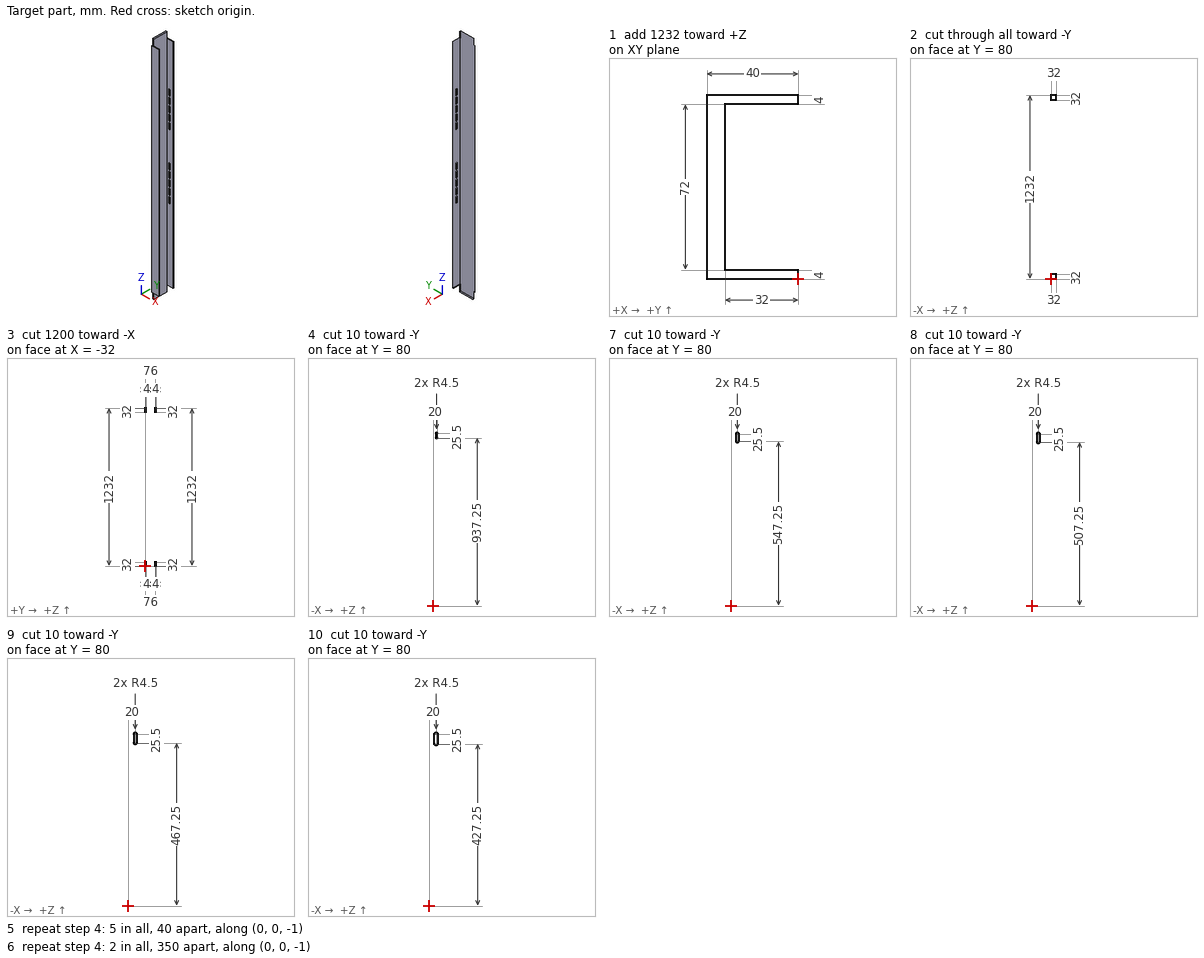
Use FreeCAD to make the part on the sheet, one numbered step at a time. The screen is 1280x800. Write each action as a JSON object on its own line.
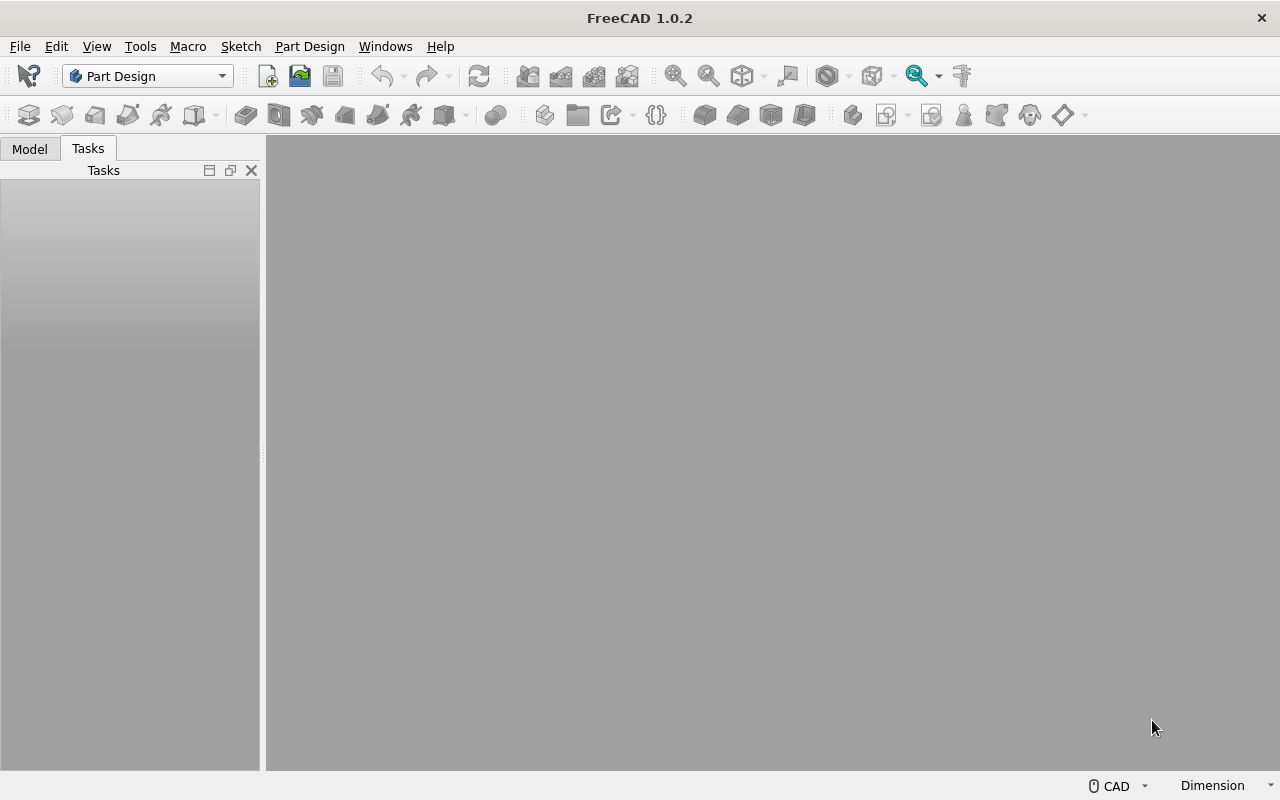
{"action": "left_click", "coordinate": [267, 76]}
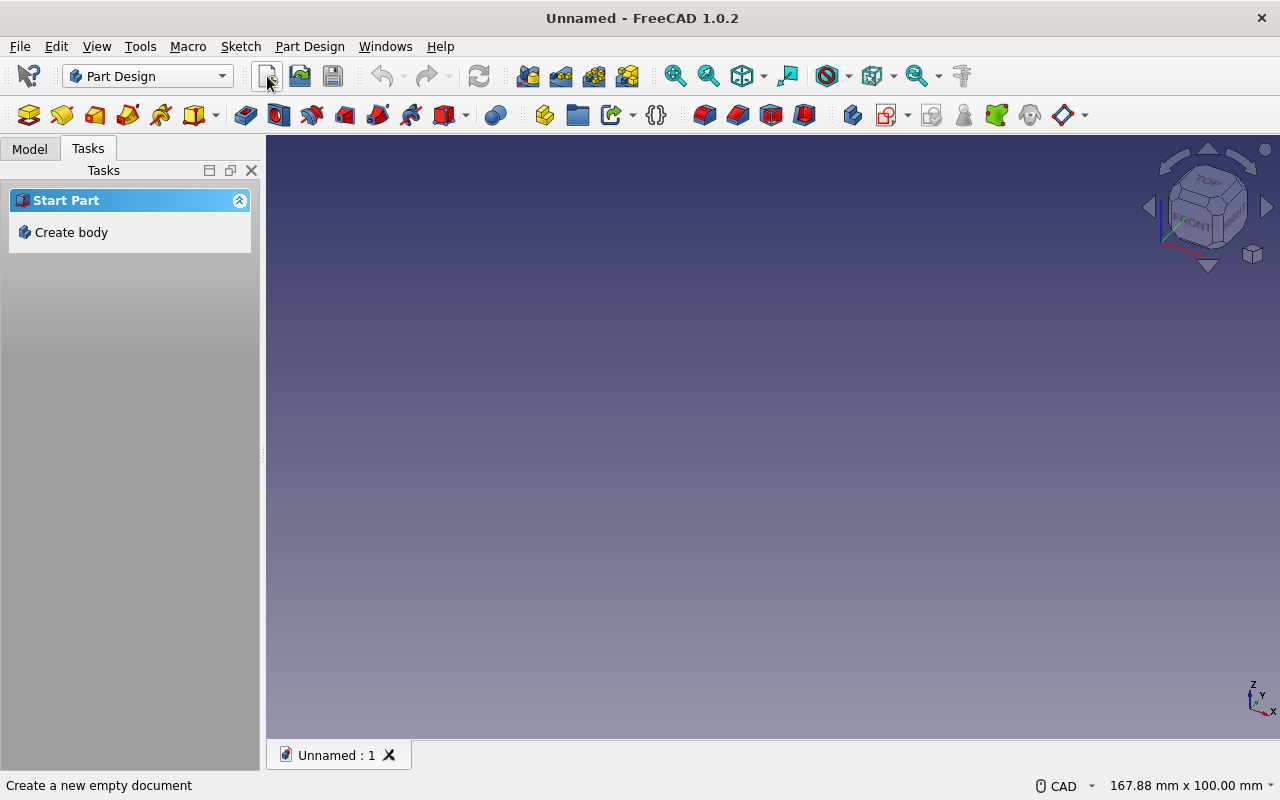
{"action": "left_click", "coordinate": [886, 116]}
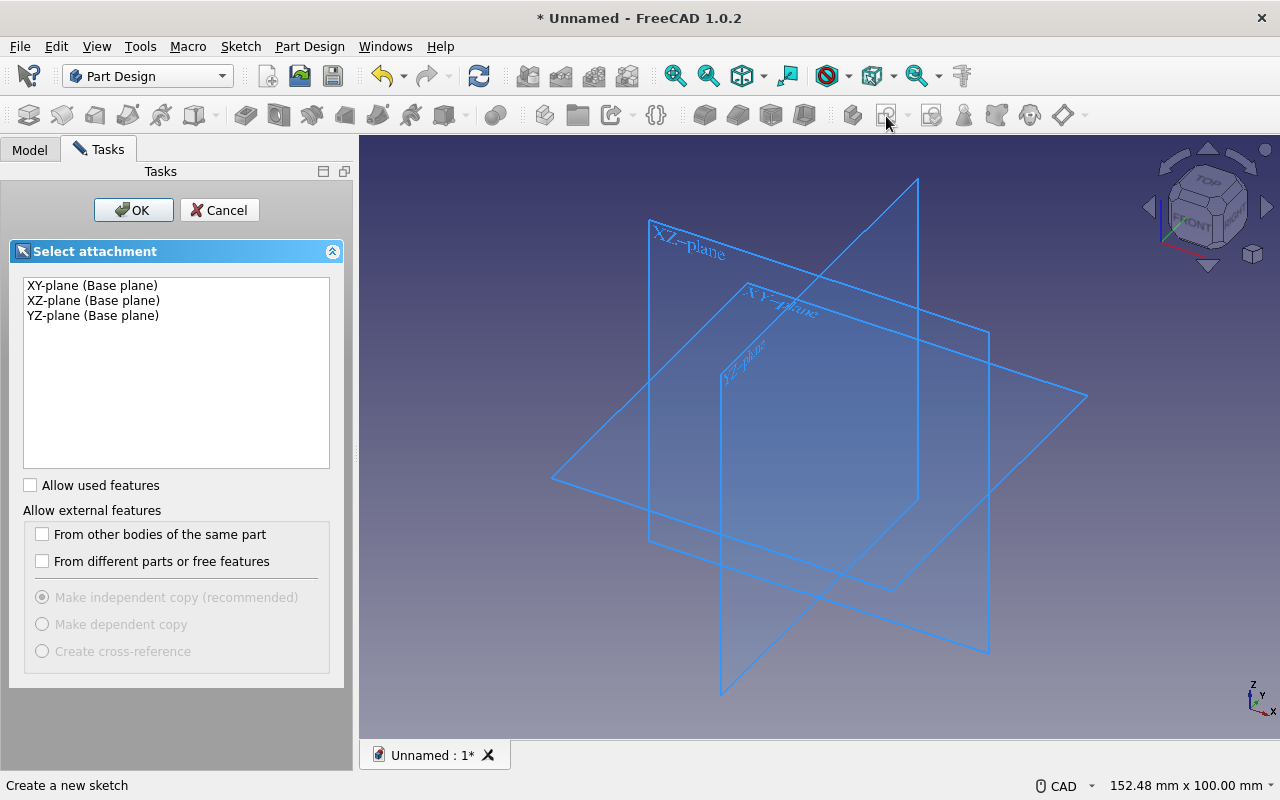
{"action": "left_click", "coordinate": [84, 286]}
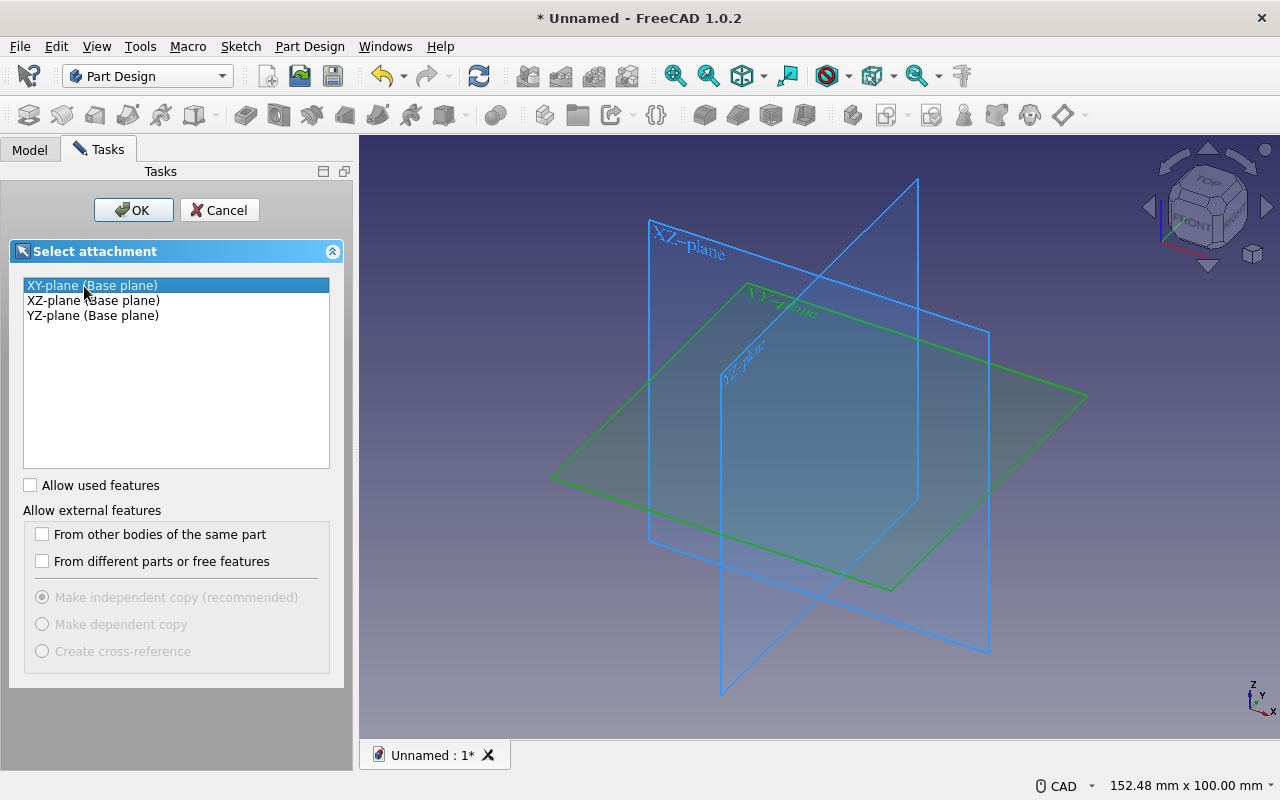
{"action": "left_click", "coordinate": [134, 210]}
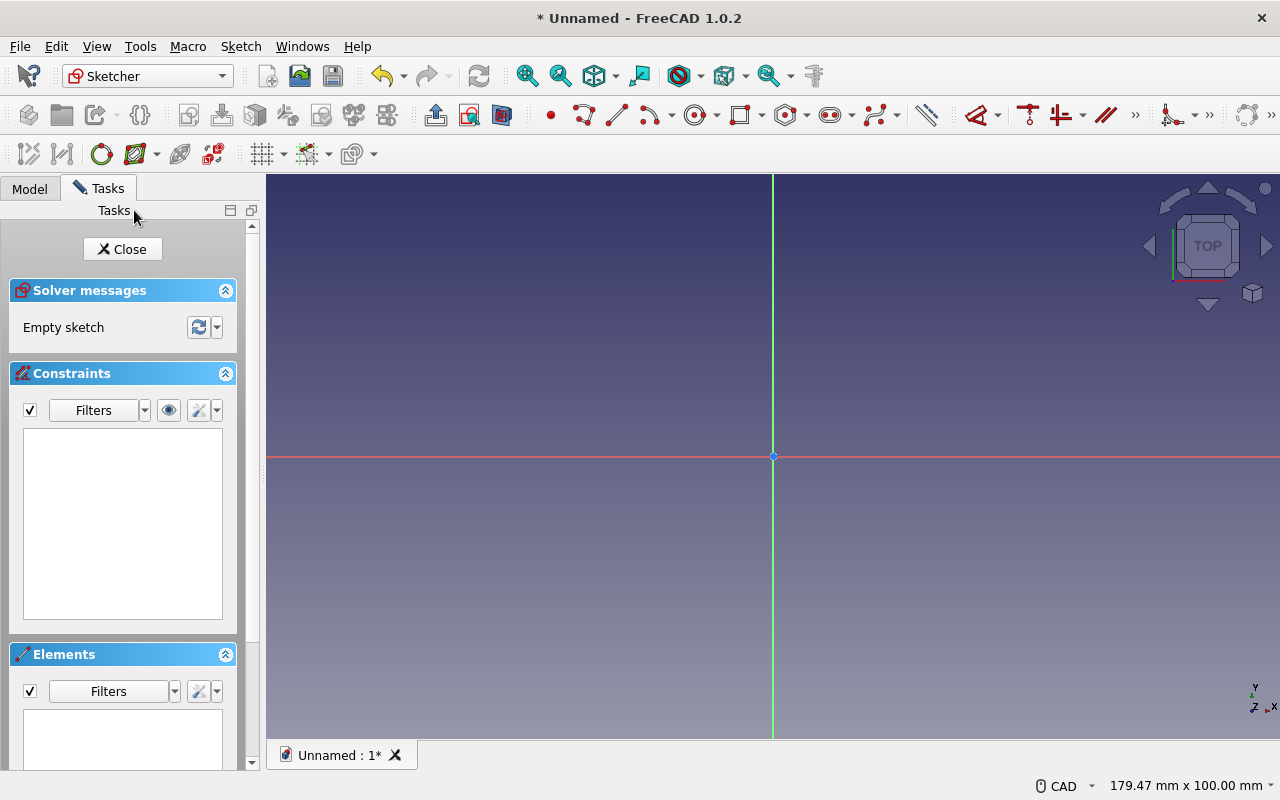
{"action": "scroll", "coordinate": [795, 711], "scroll_direction": "down", "scroll_amount": 2}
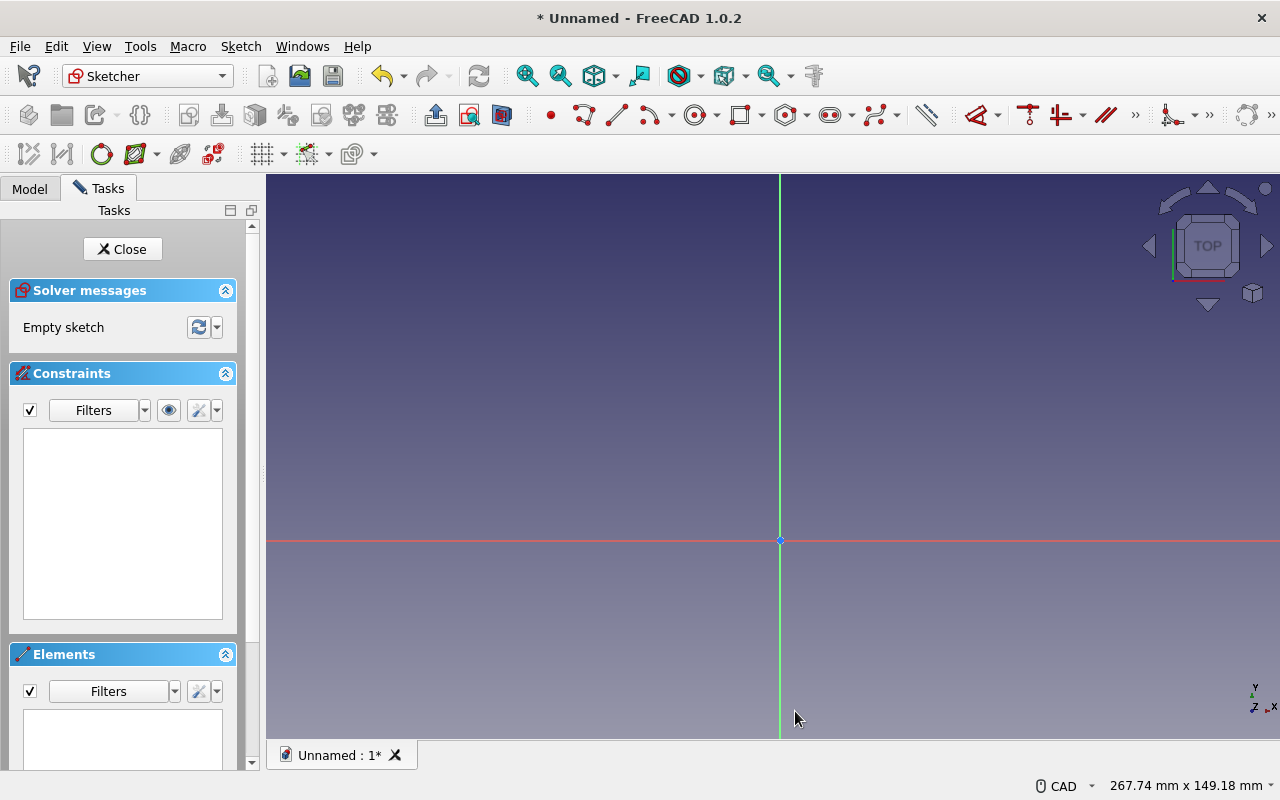
{"action": "left_click", "coordinate": [584, 116]}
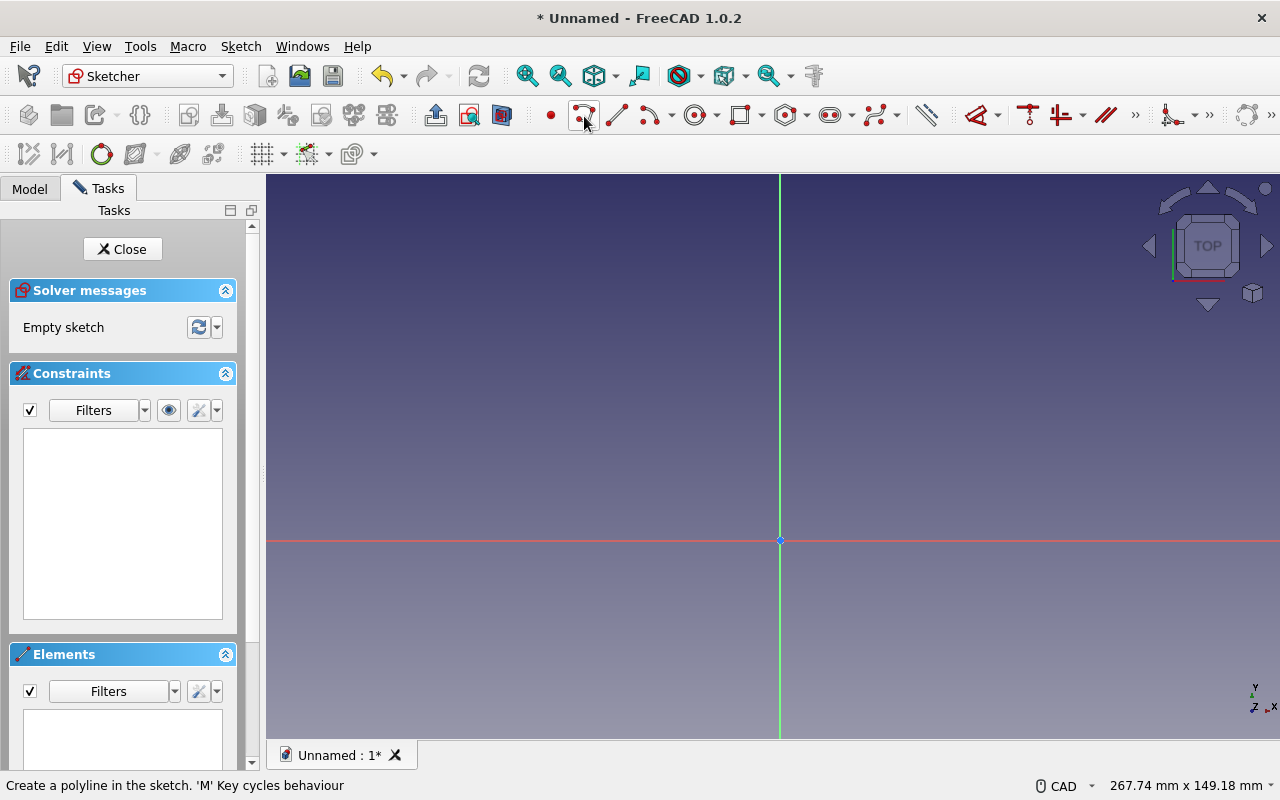
{"action": "left_click", "coordinate": [780, 541]}
{"action": "left_click", "coordinate": [771, 526]}
{"action": "left_click", "coordinate": [659, 526]}
{"action": "left_click", "coordinate": [659, 253]}
{"action": "left_click", "coordinate": [780, 253]}
{"action": "left_click", "coordinate": [771, 238]}
{"action": "left_click", "coordinate": [629, 238]}
{"action": "left_click", "coordinate": [629, 532]}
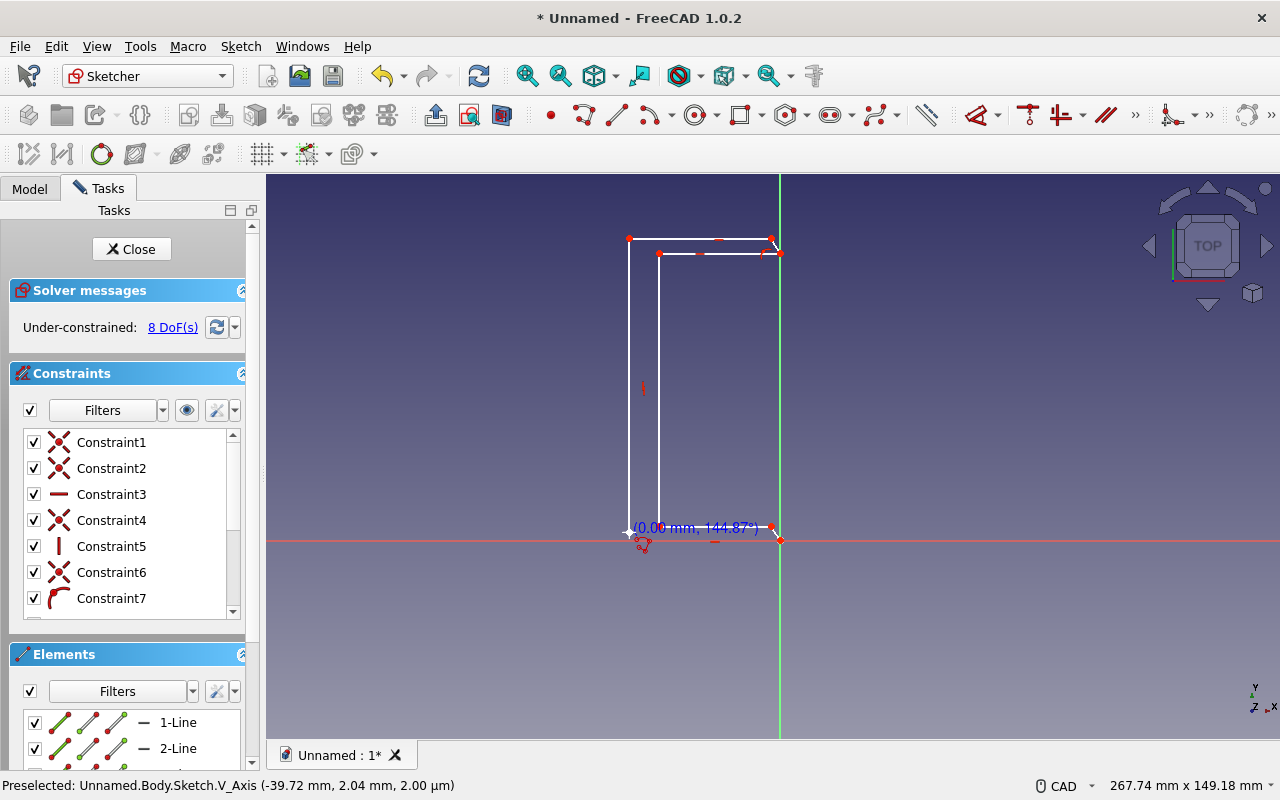
{"action": "scroll", "coordinate": [780, 541], "scroll_direction": "up", "scroll_amount": 4}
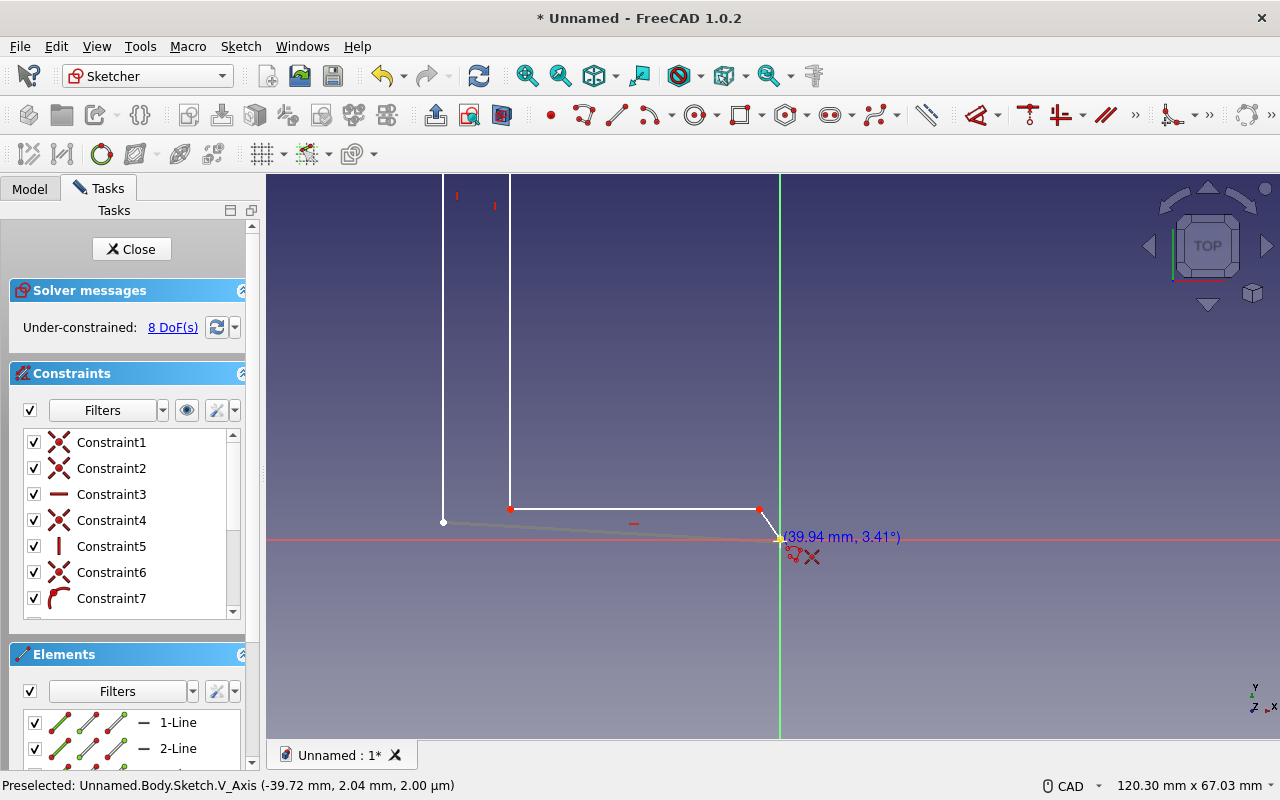
{"action": "left_click", "coordinate": [780, 540]}
{"action": "key", "text": "Escape"}
{"action": "key", "text": "Escape"}